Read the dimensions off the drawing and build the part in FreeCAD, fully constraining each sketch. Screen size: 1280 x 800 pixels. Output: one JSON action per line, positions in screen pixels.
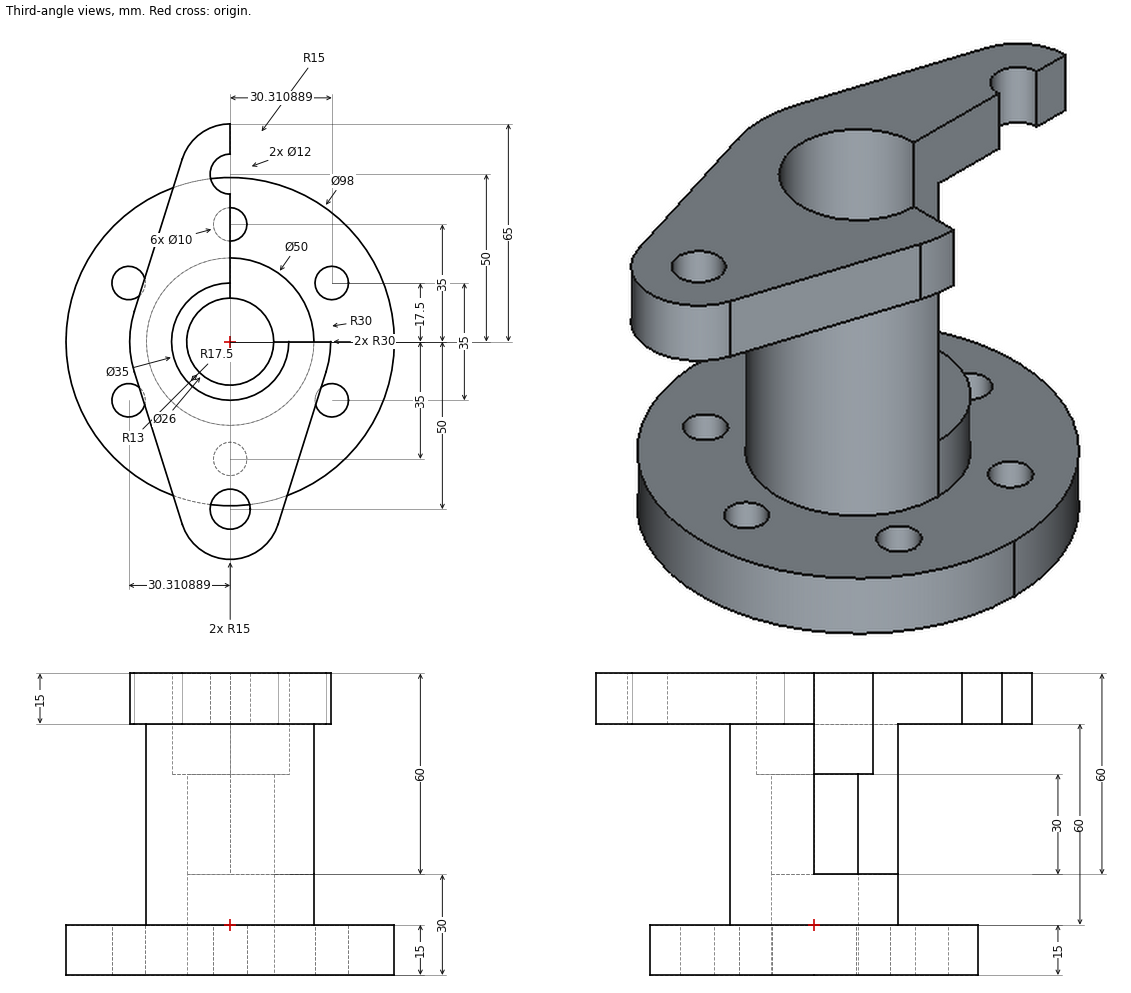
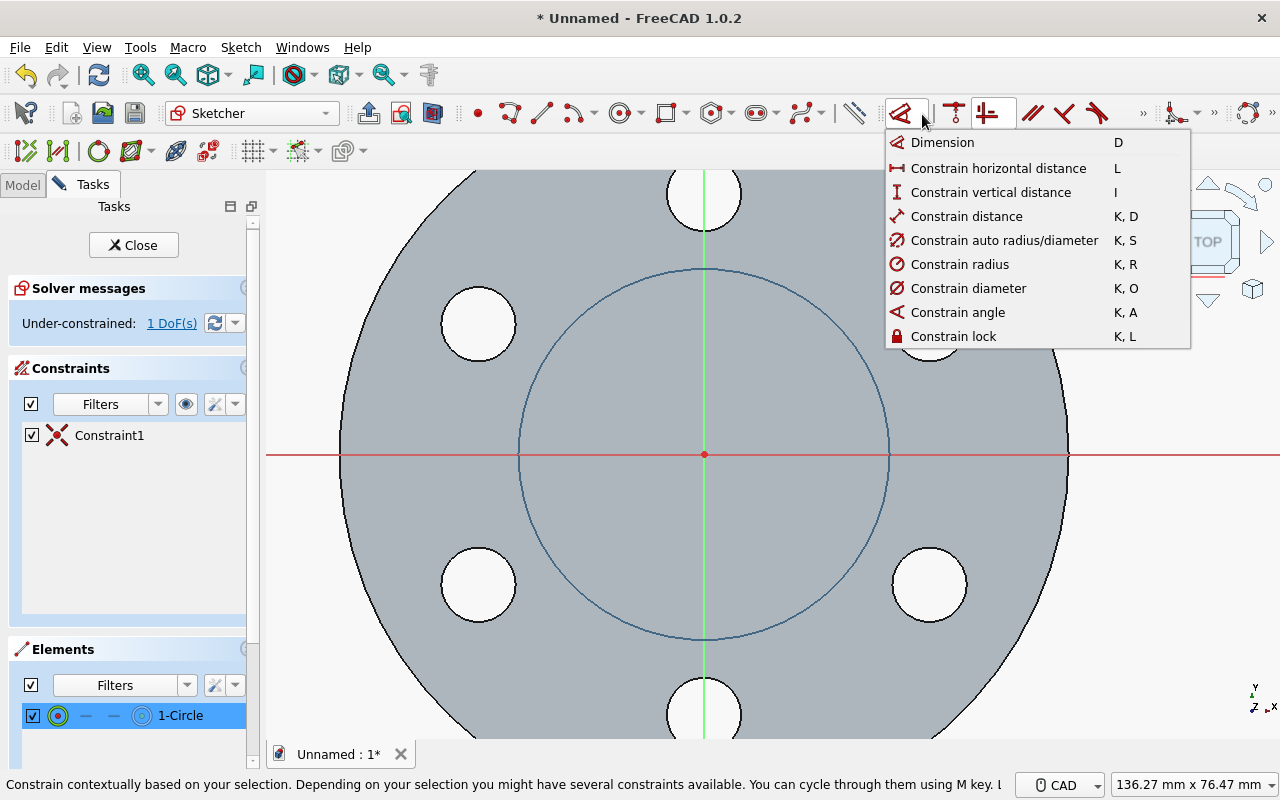
{"action": "left_click", "coordinate": [1038, 288]}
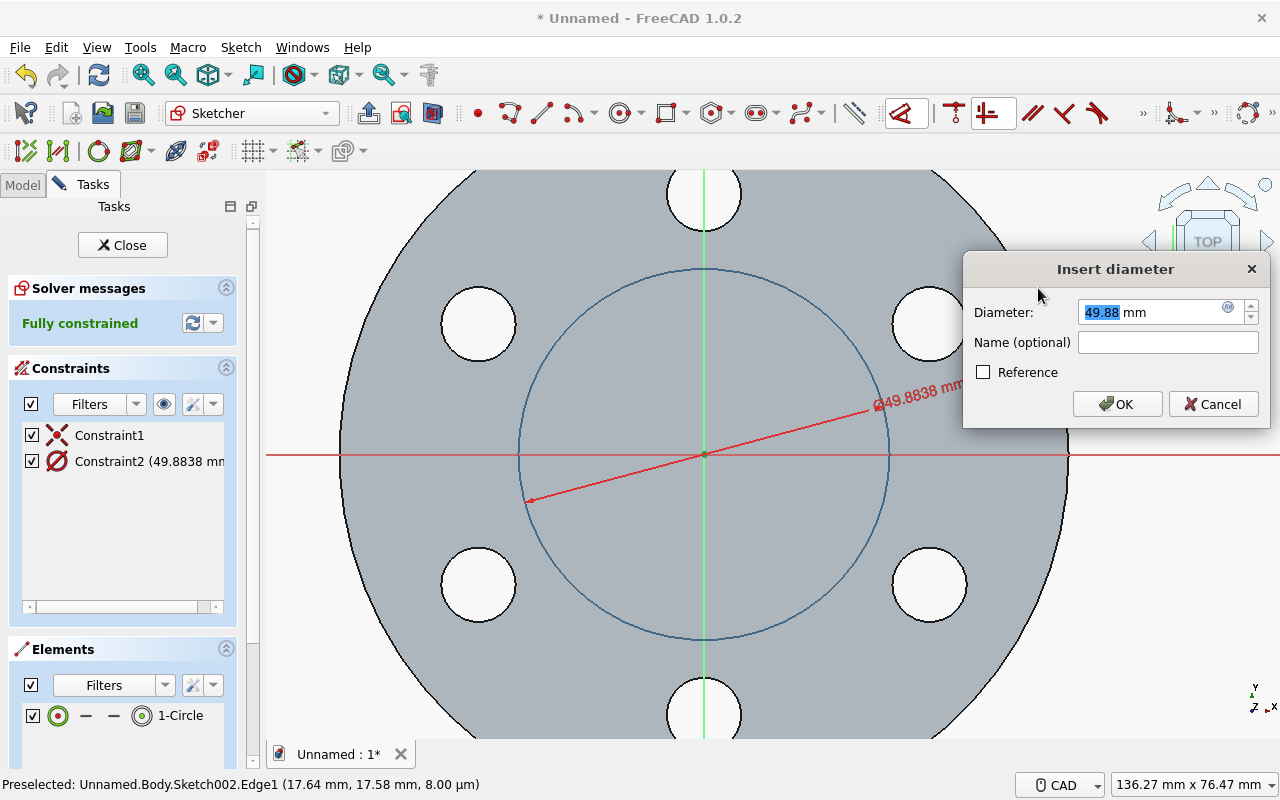
{"action": "type", "text": "50"}
{"action": "key", "text": "Return"}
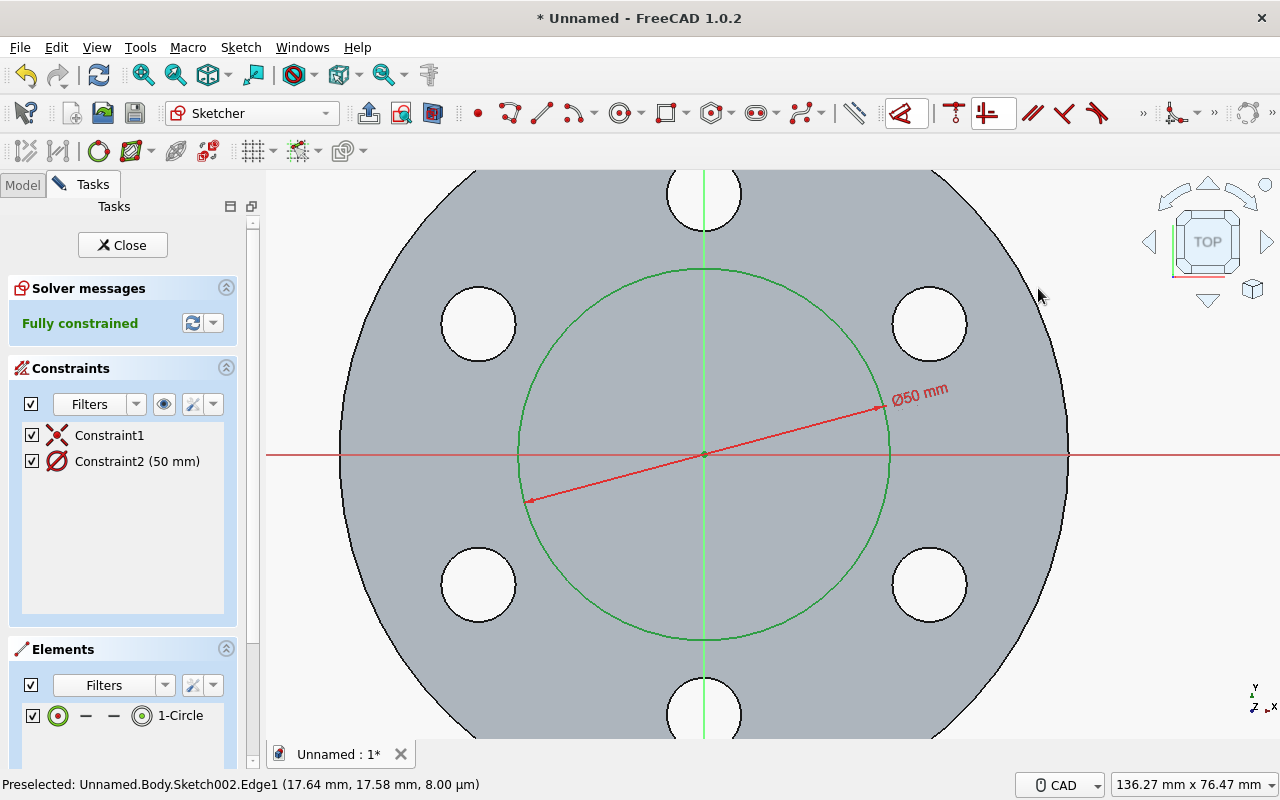
{"action": "left_click", "coordinate": [123, 245]}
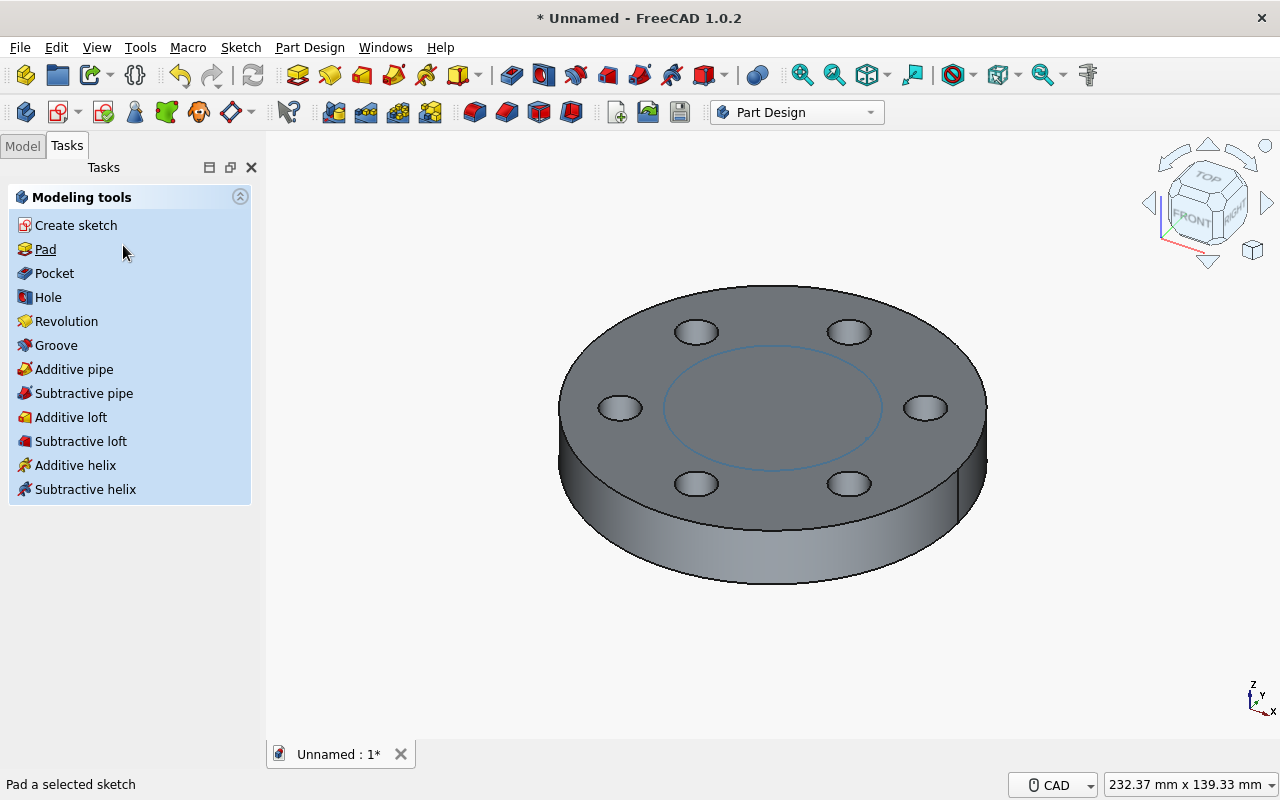
{"action": "left_click", "coordinate": [298, 76]}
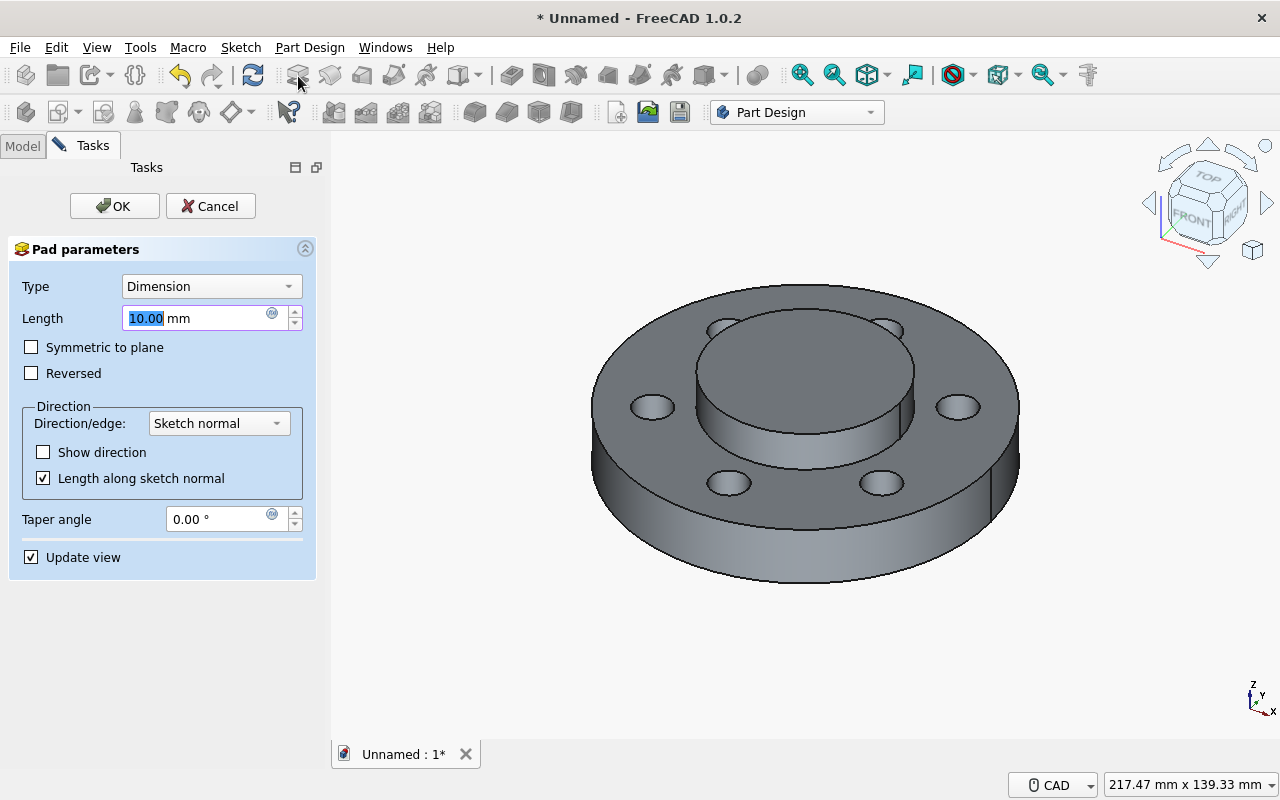
{"action": "type", "text": "60"}
{"action": "key", "text": "Tab"}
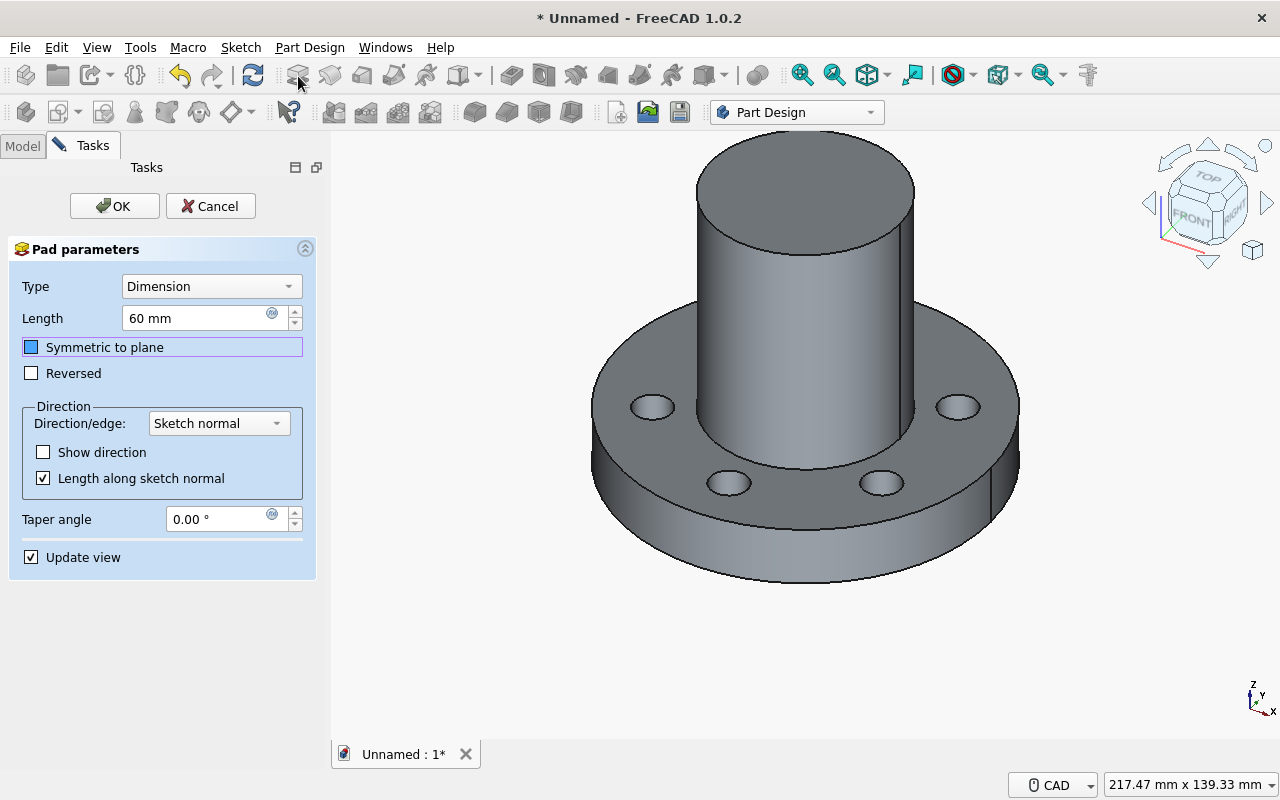
{"action": "left_click", "coordinate": [115, 206]}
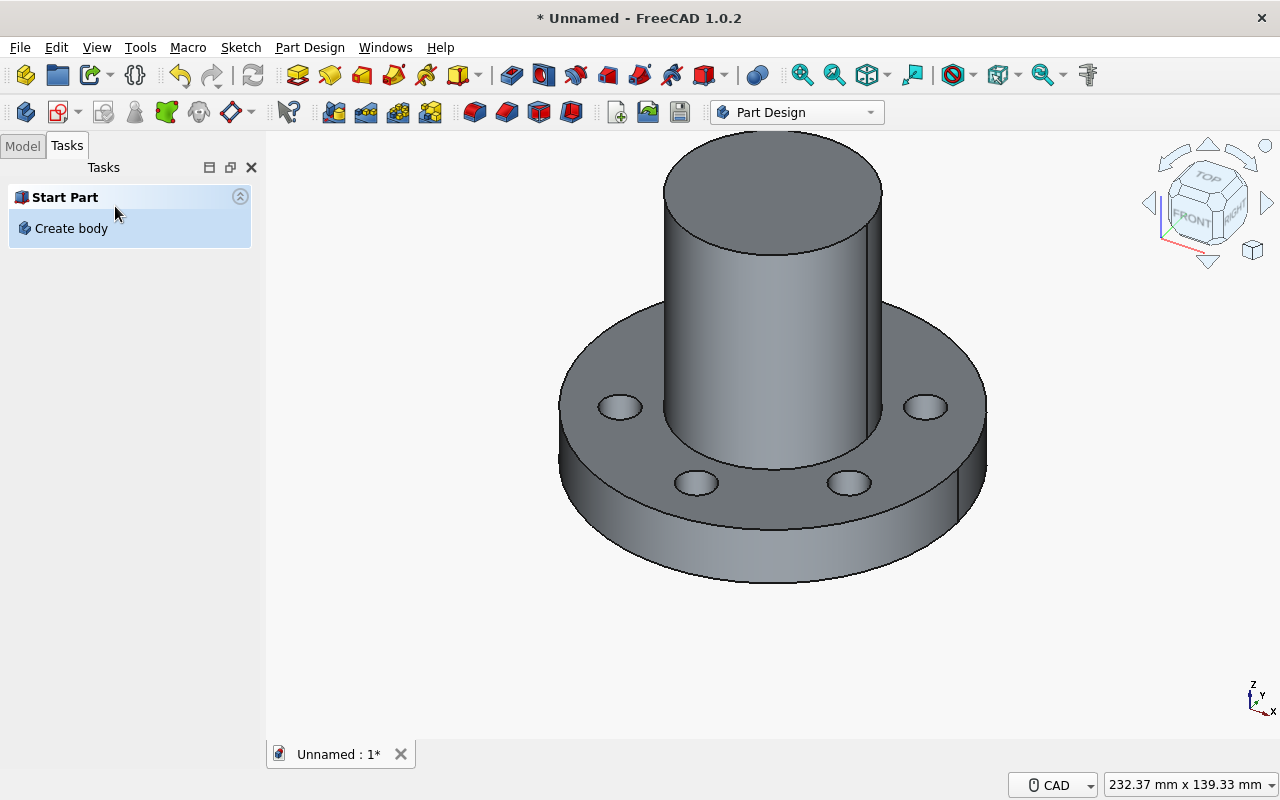
{"action": "left_click", "coordinate": [804, 76]}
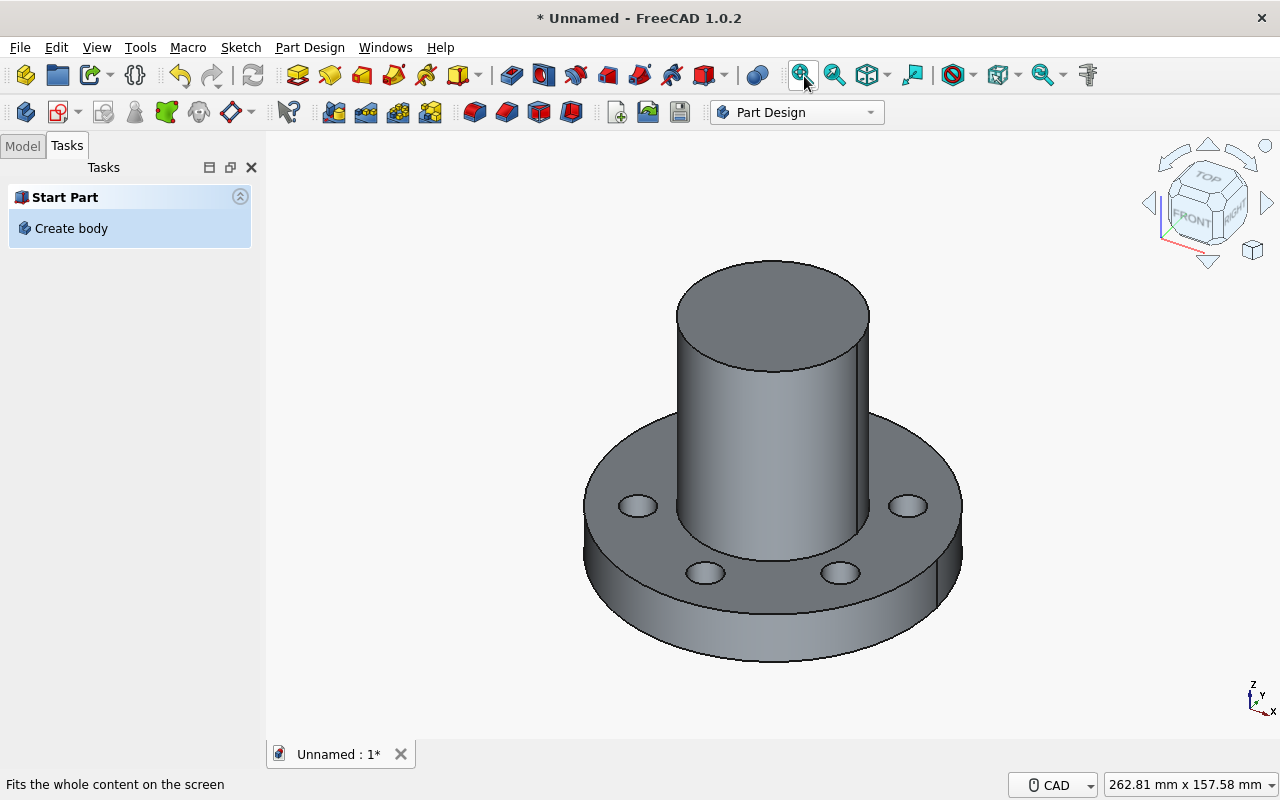
{"action": "left_click", "coordinate": [773, 315]}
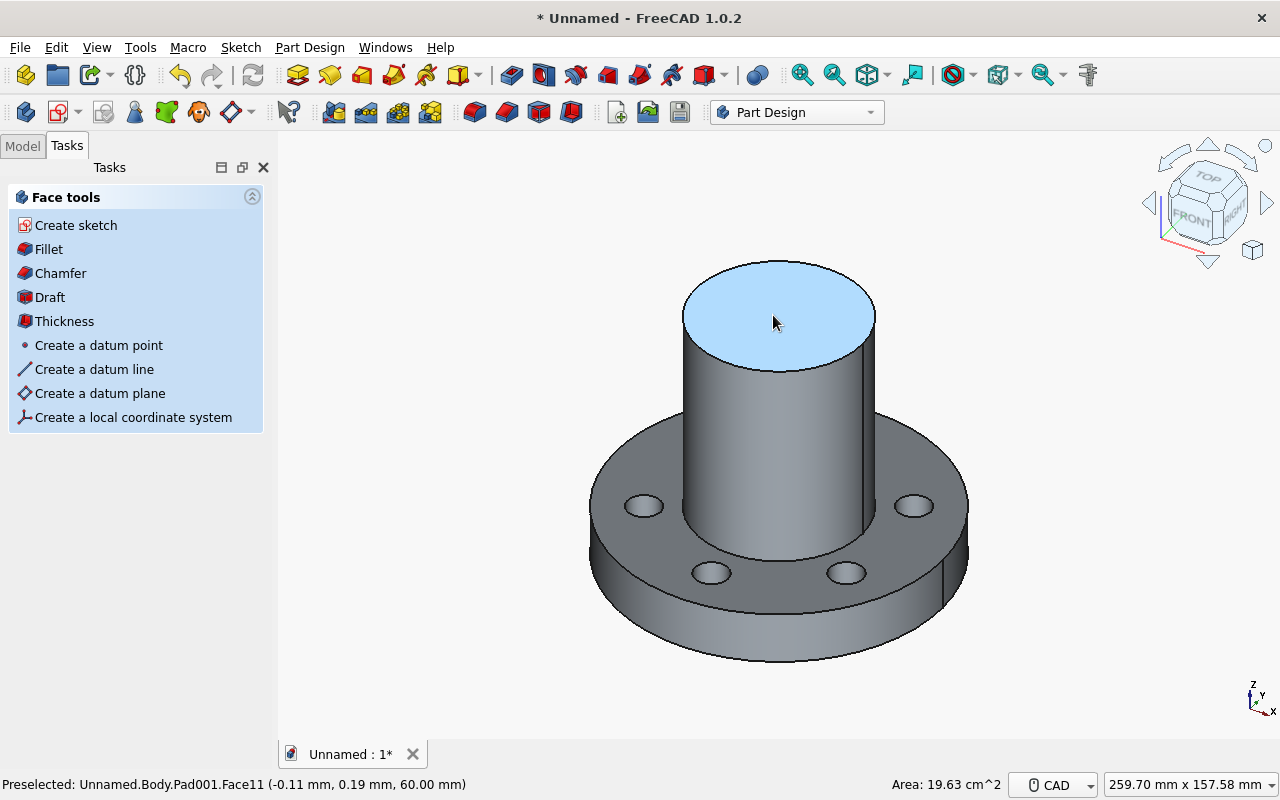
{"action": "left_click", "coordinate": [58, 112]}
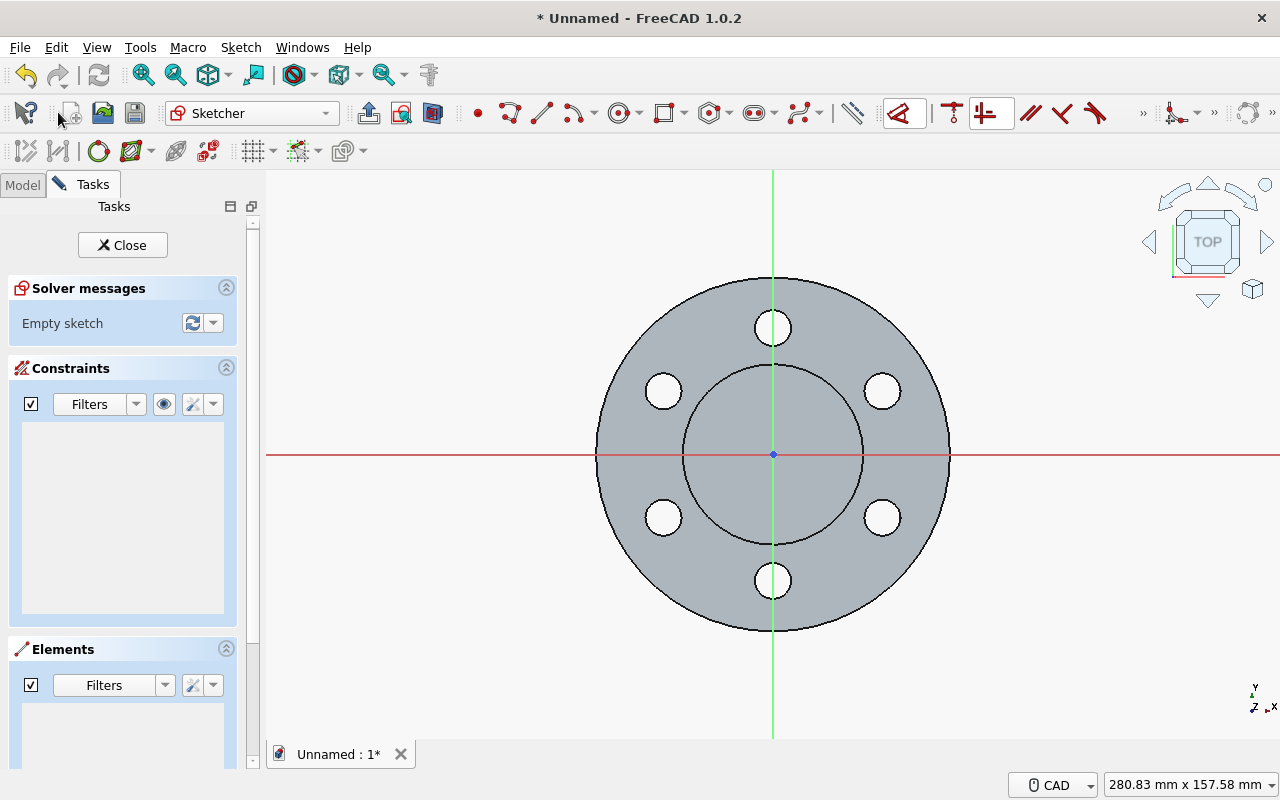
{"action": "scroll", "coordinate": [395, 455], "scroll_direction": "down", "scroll_amount": 1}